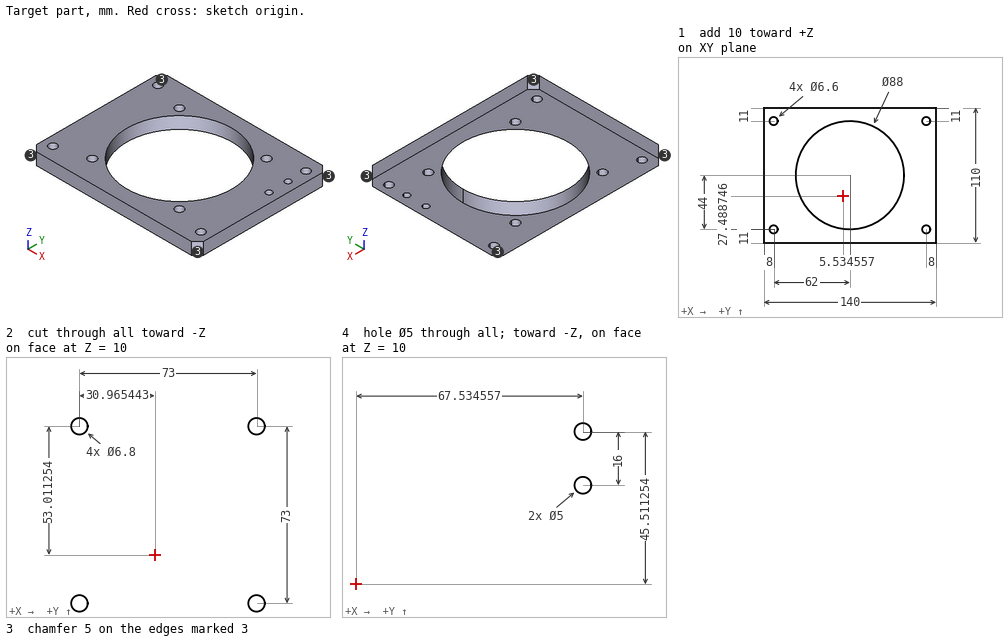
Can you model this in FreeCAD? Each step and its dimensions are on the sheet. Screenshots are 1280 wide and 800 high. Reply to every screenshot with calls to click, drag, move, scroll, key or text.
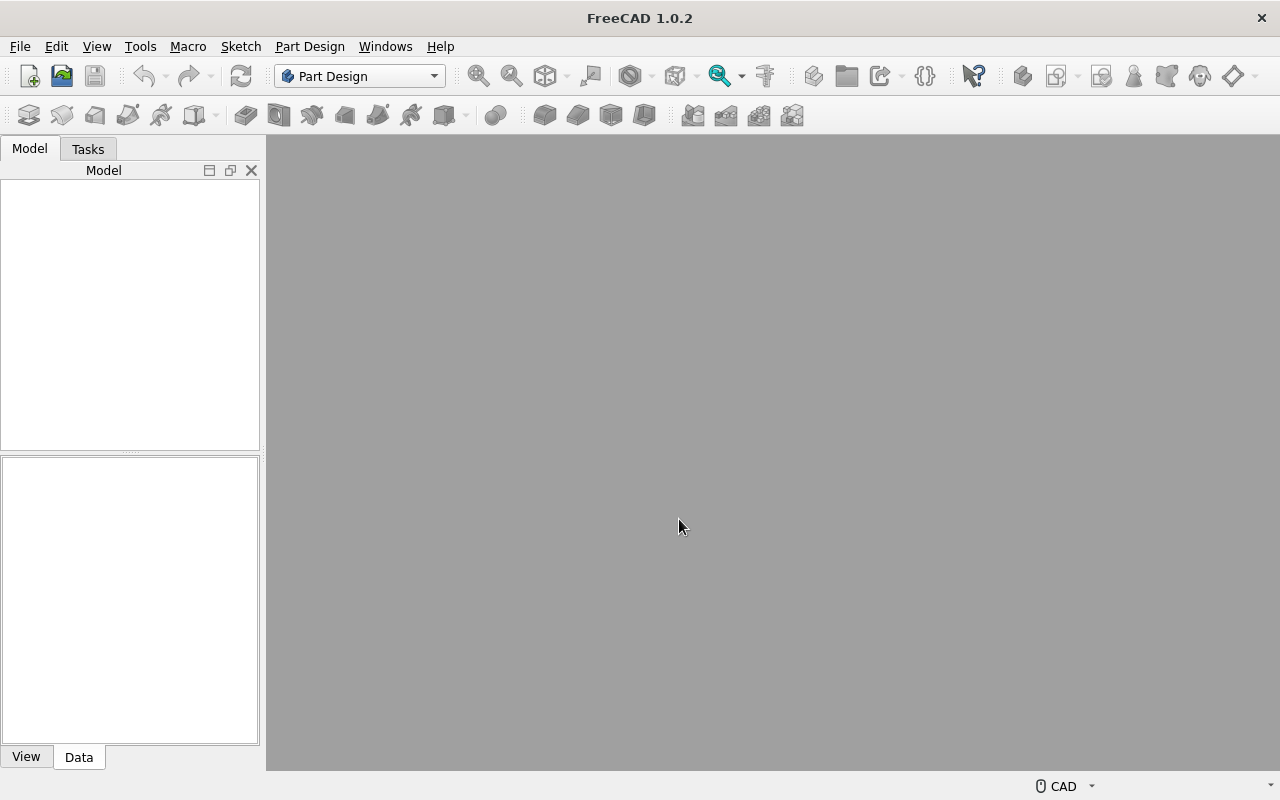
click(29, 76)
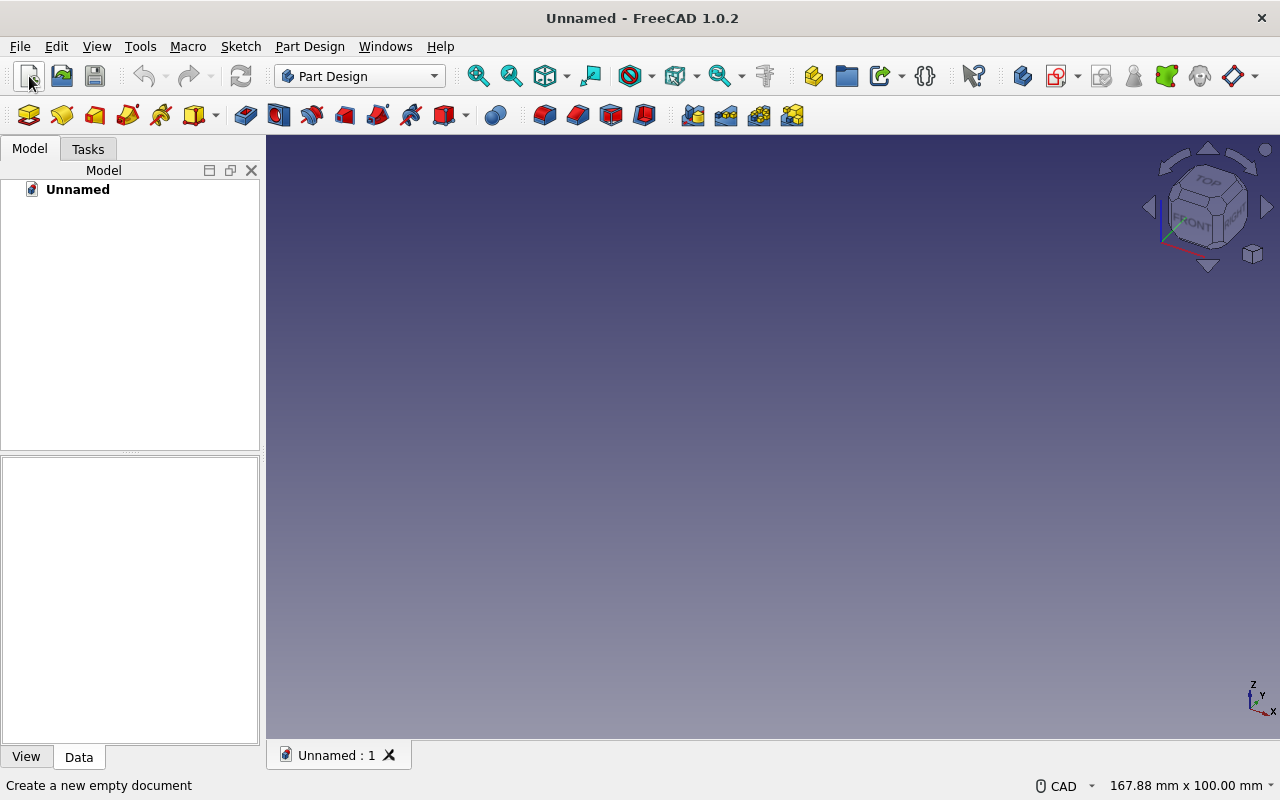
click(1056, 76)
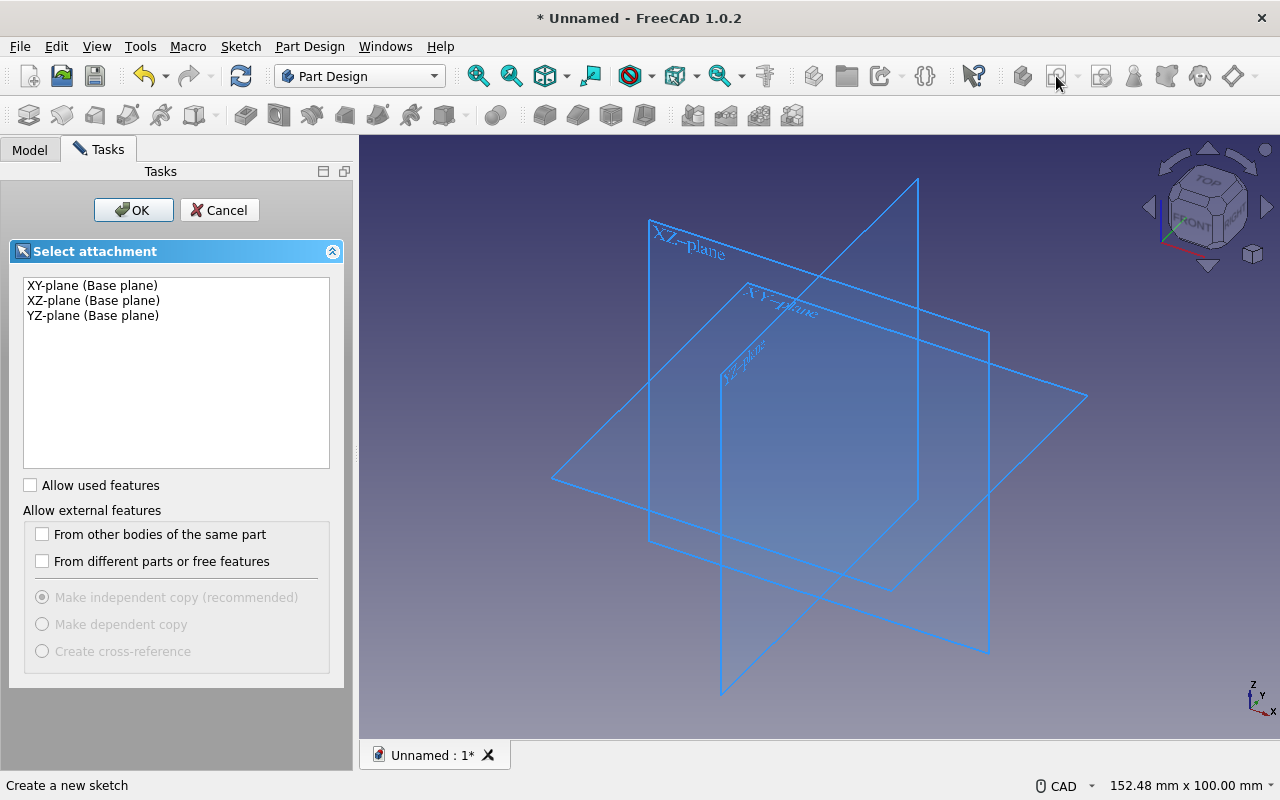
click(84, 286)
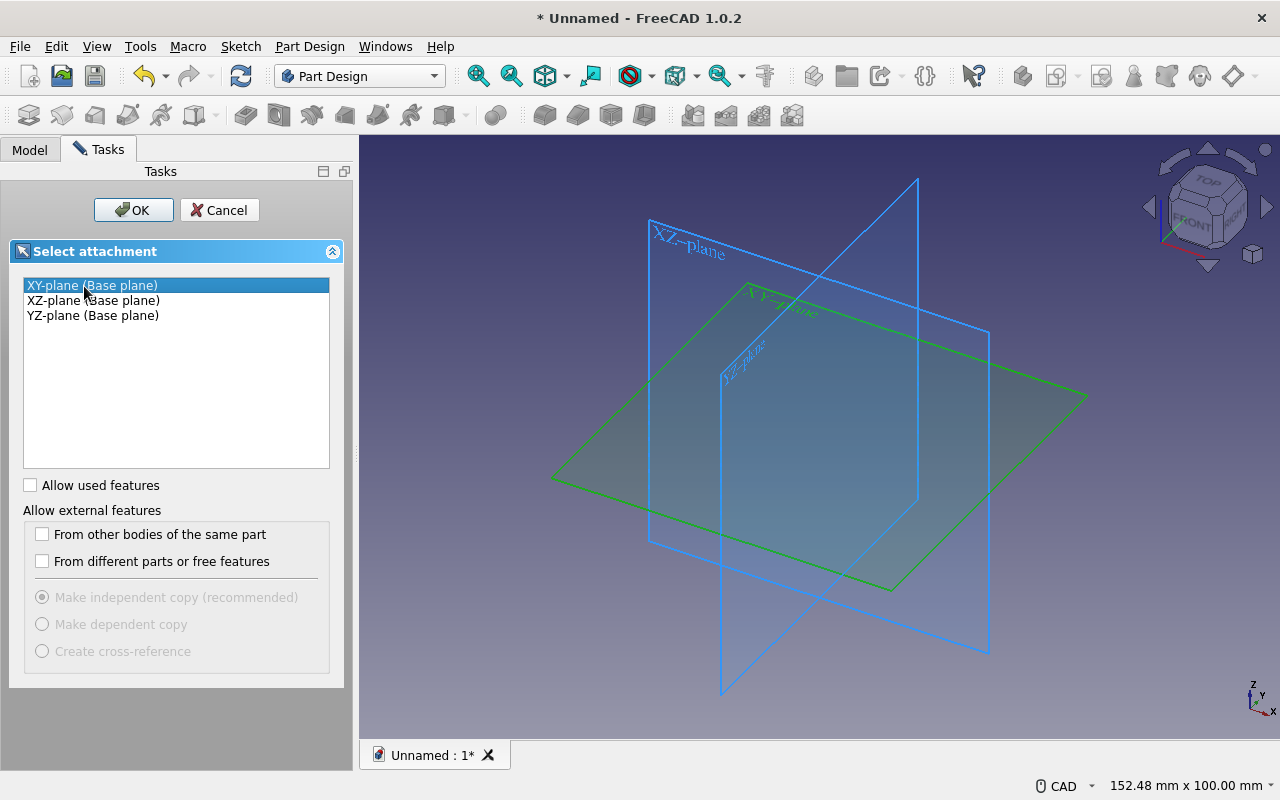
click(134, 210)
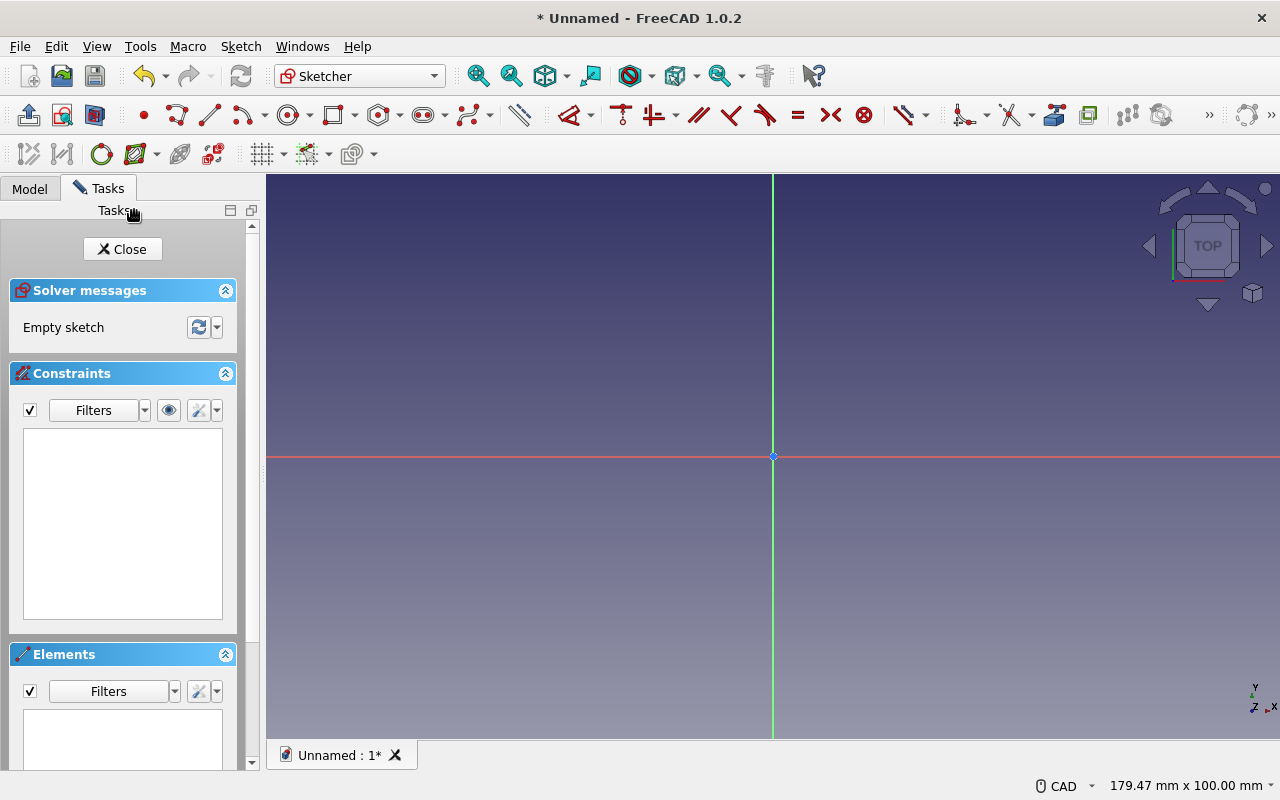
scroll(583, 570, down, 3)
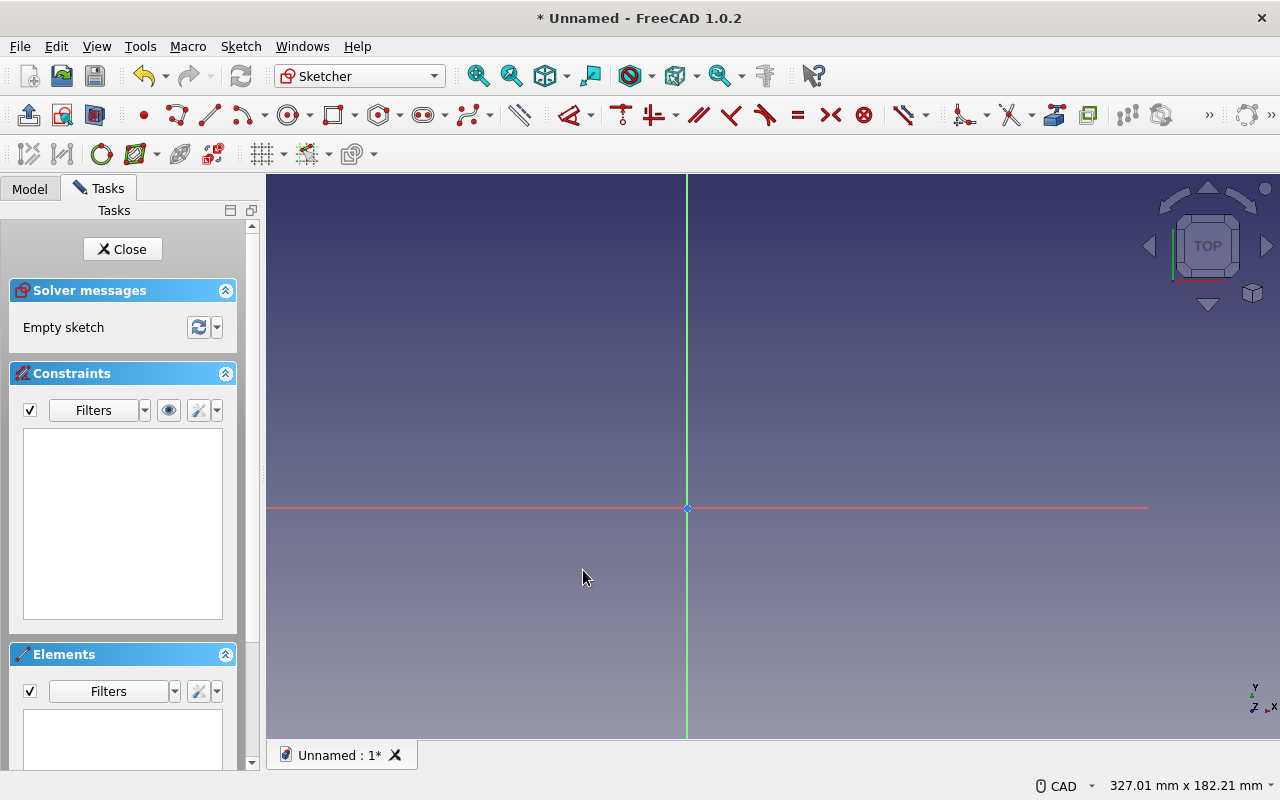
click(332, 116)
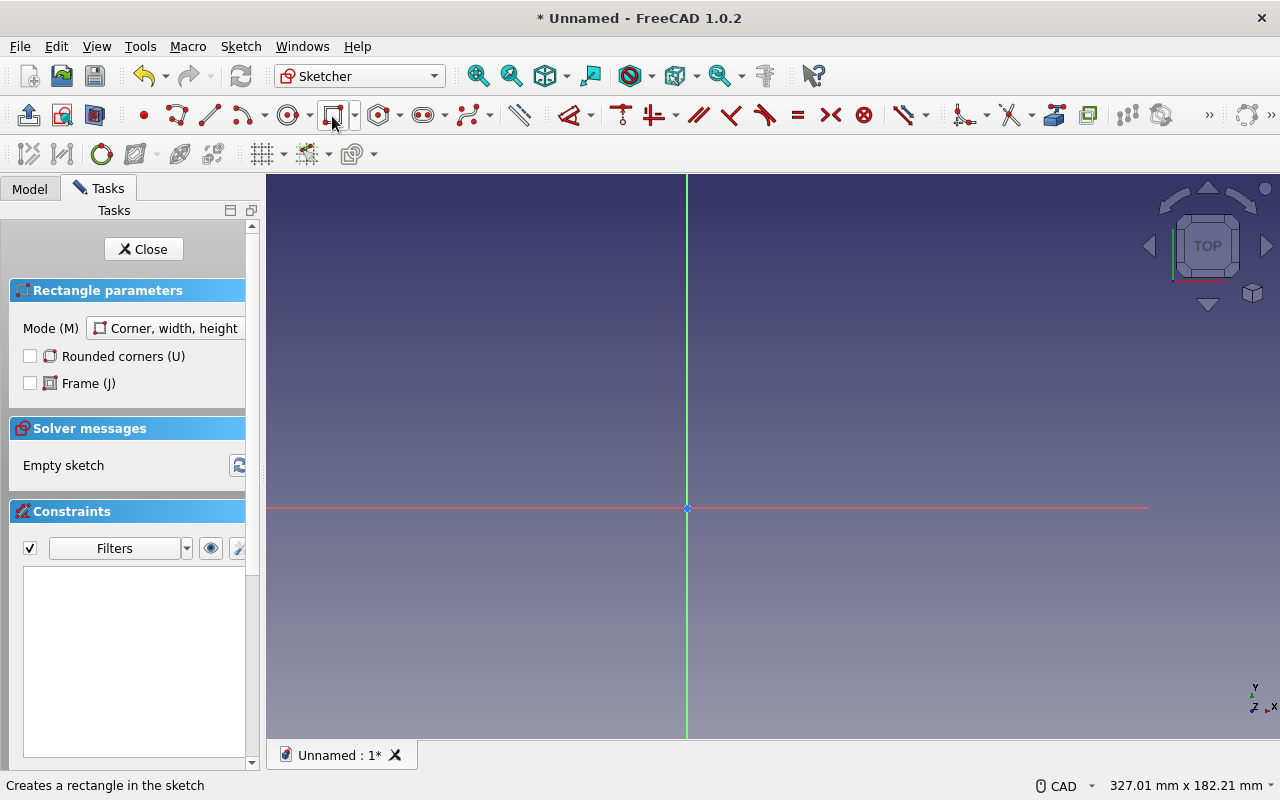
click(488, 286)
move(922, 627)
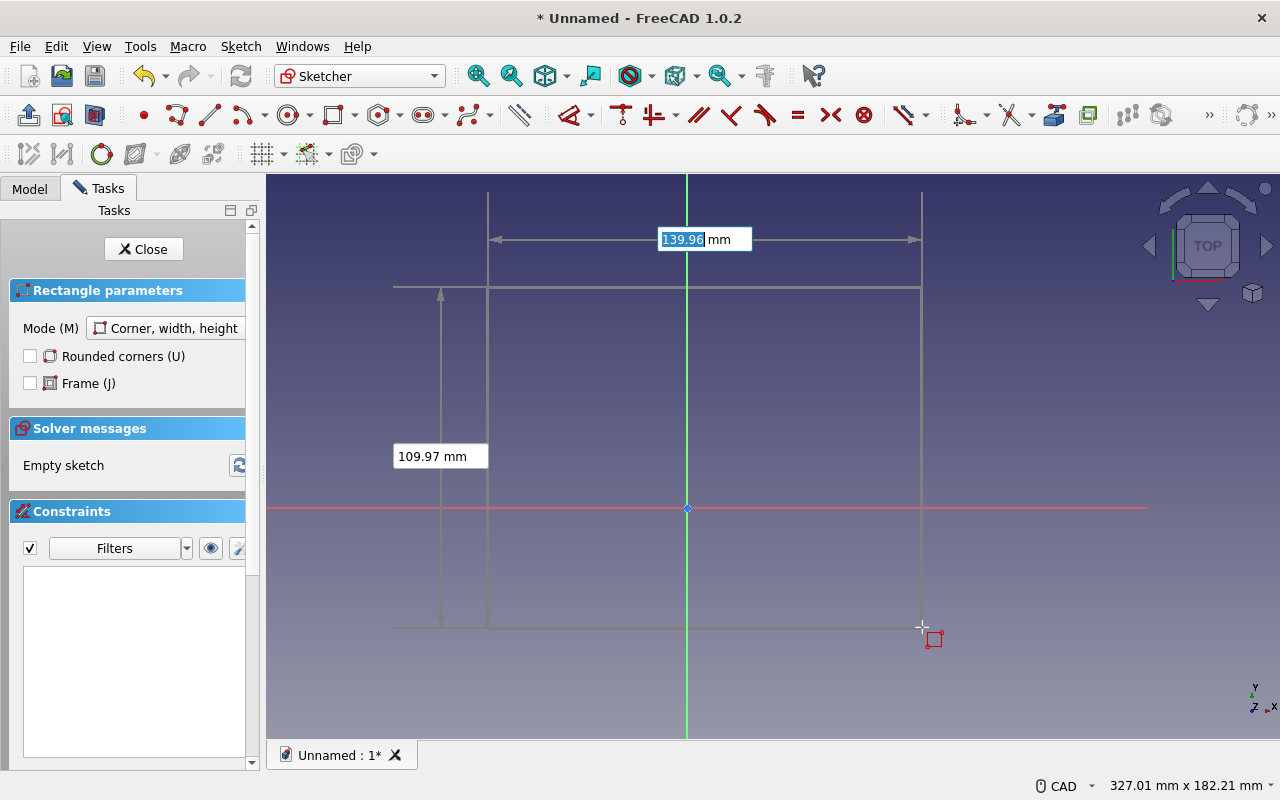
text(140)
key(Tab)
text(110)
key(Return)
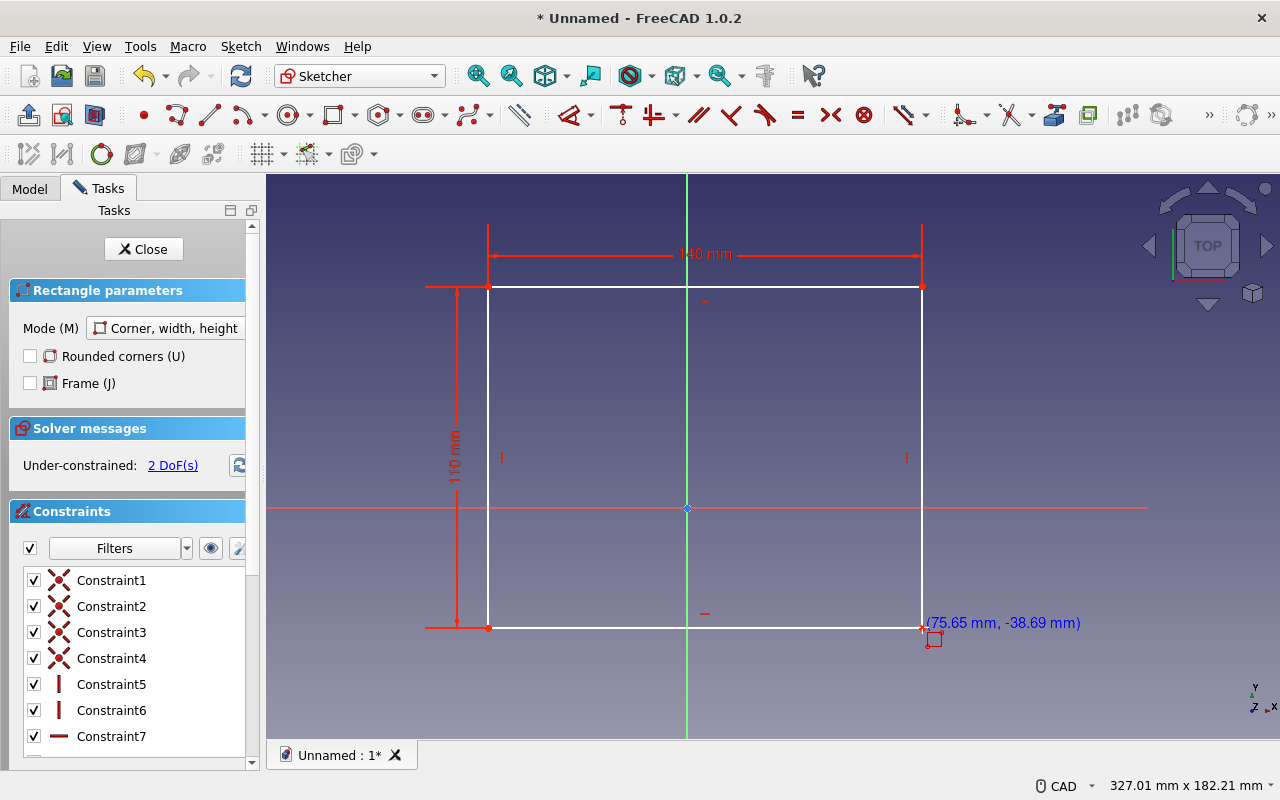
click(288, 116)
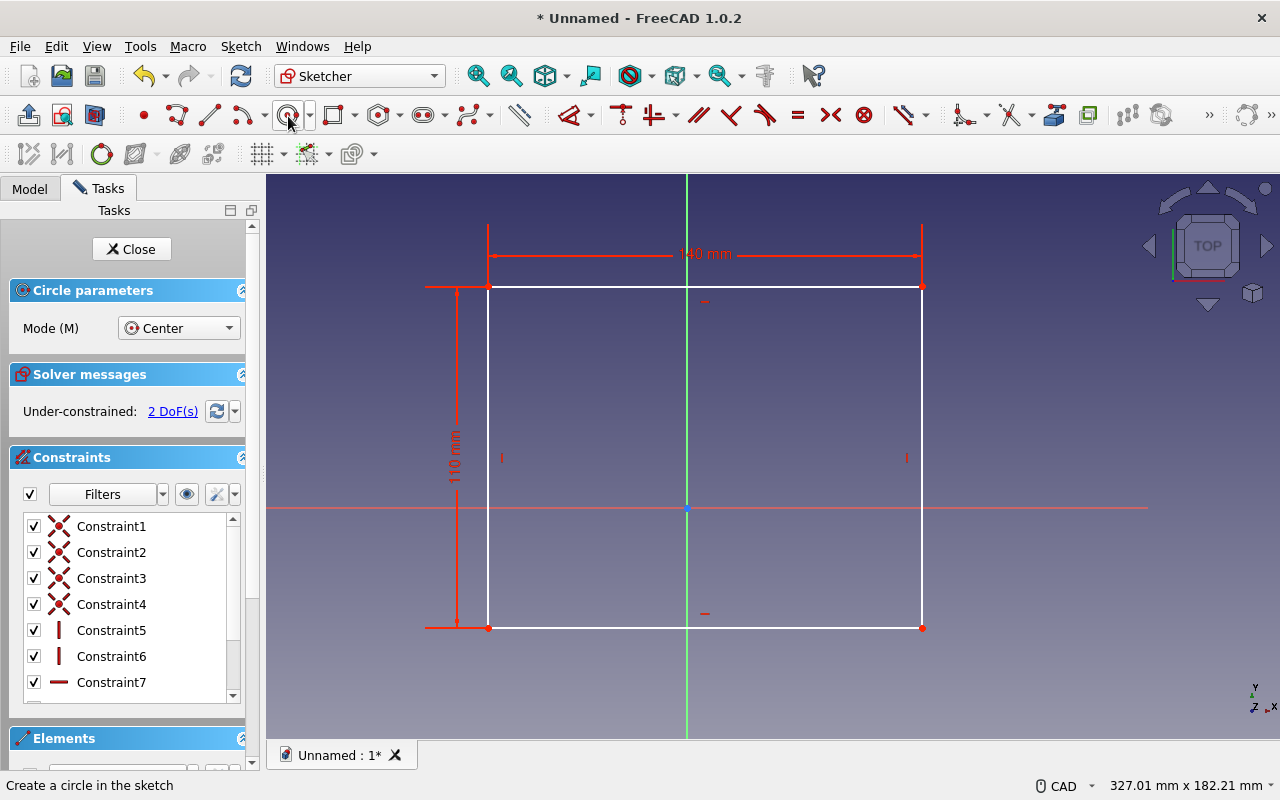
scroll(512, 593, up, 4)